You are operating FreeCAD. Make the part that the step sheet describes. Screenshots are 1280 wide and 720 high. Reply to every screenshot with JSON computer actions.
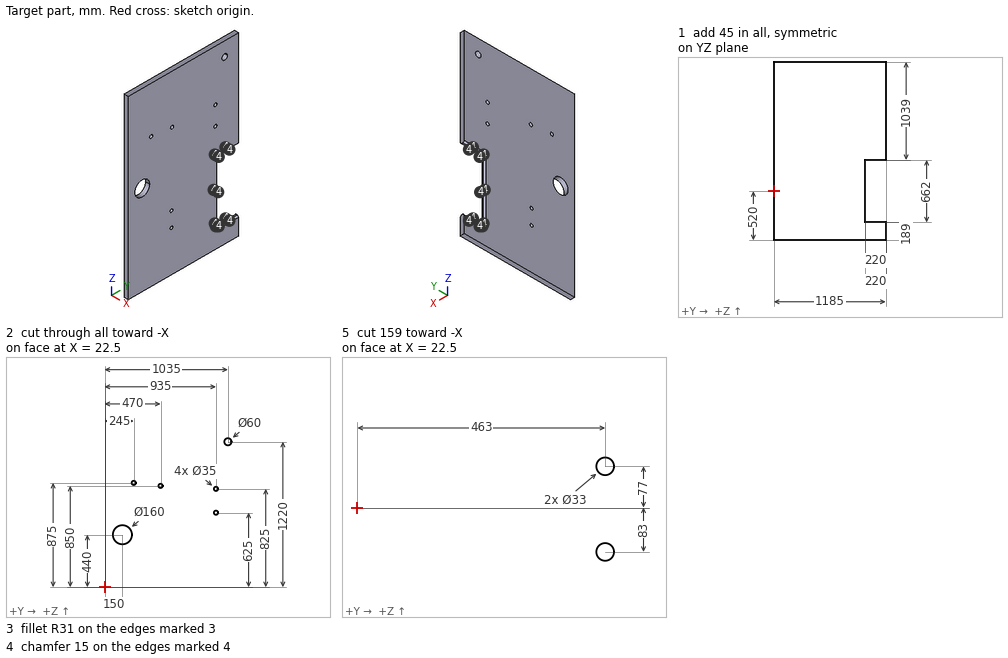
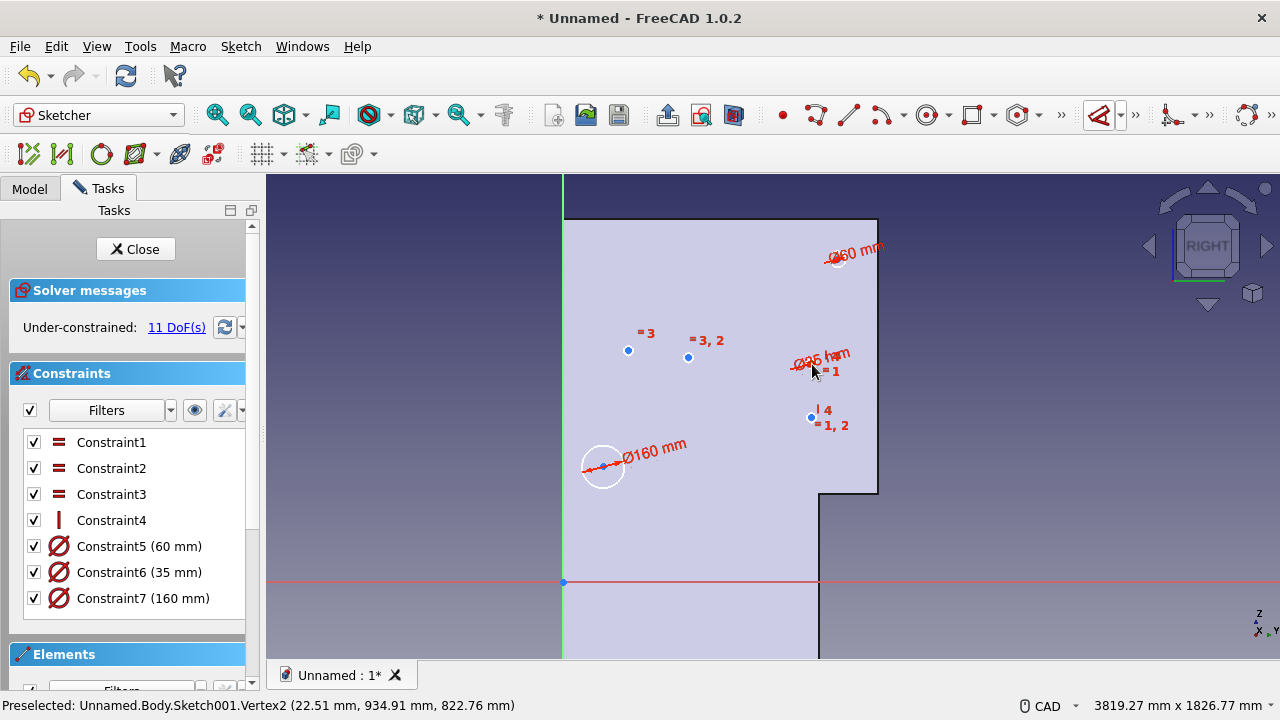
{"action": "left_click", "coordinate": [1120, 116]}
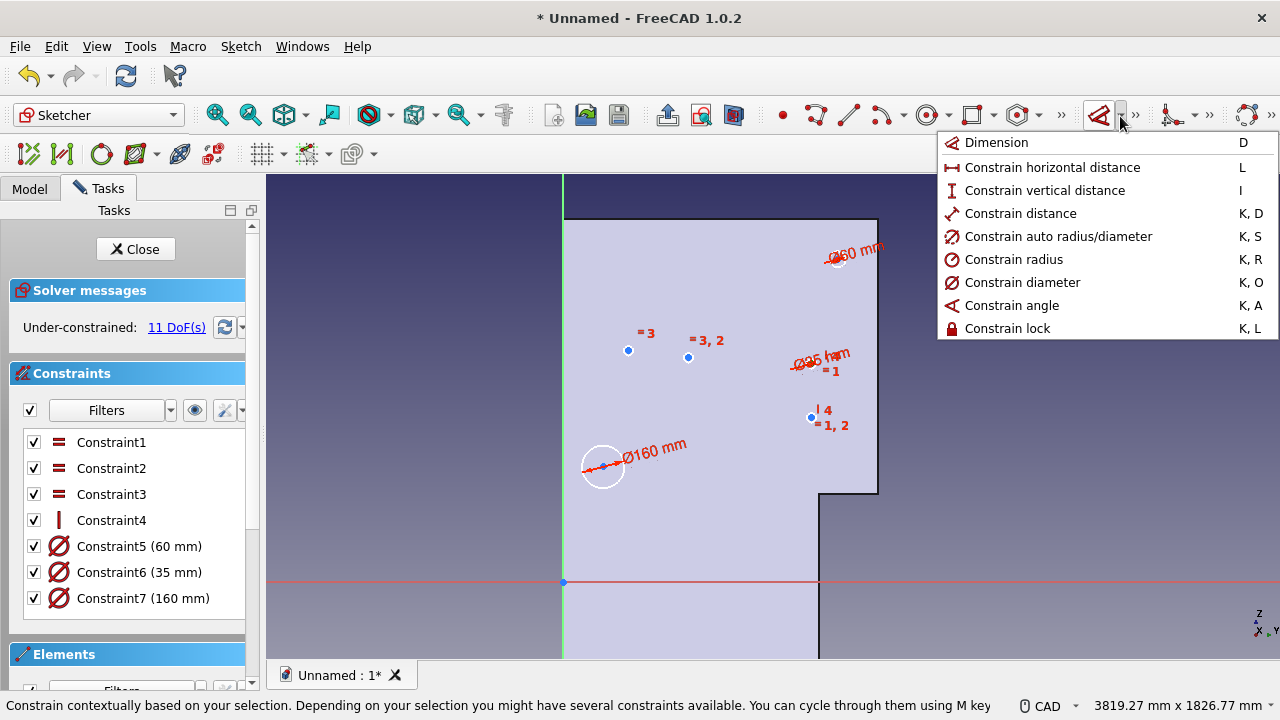
{"action": "left_click", "coordinate": [1108, 168]}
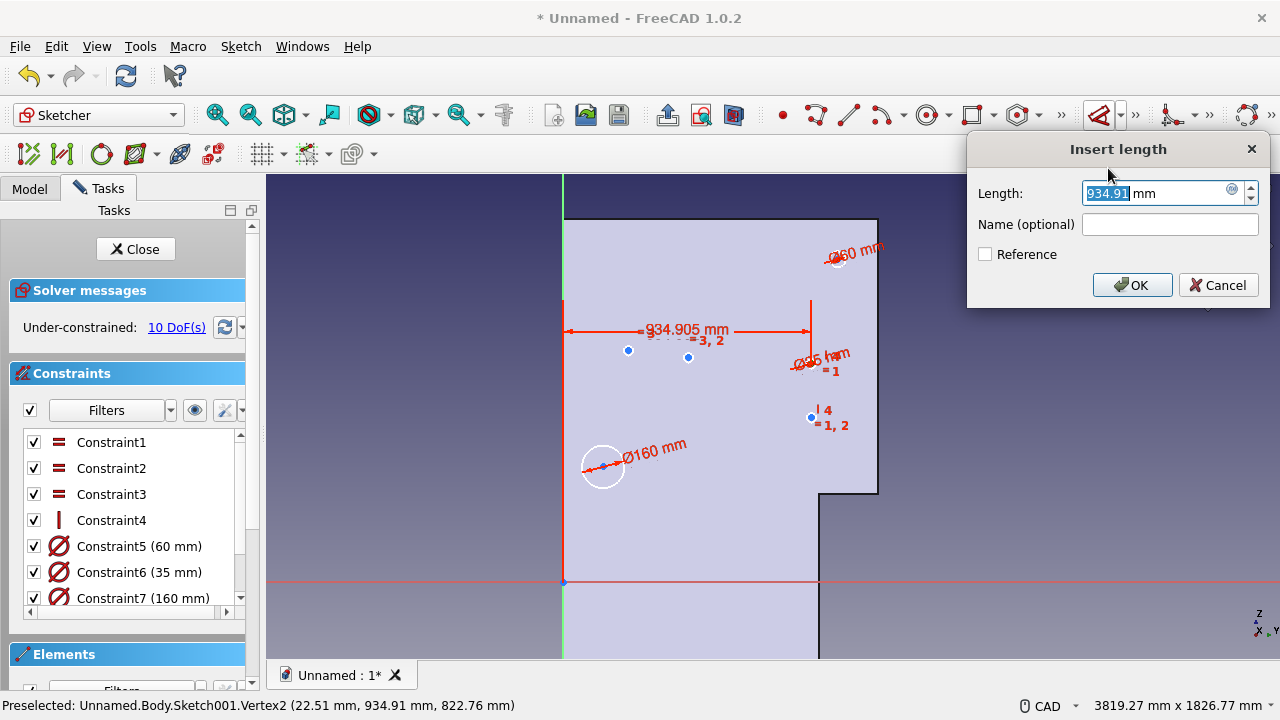
{"action": "type", "text": "935"}
{"action": "key", "text": "Return"}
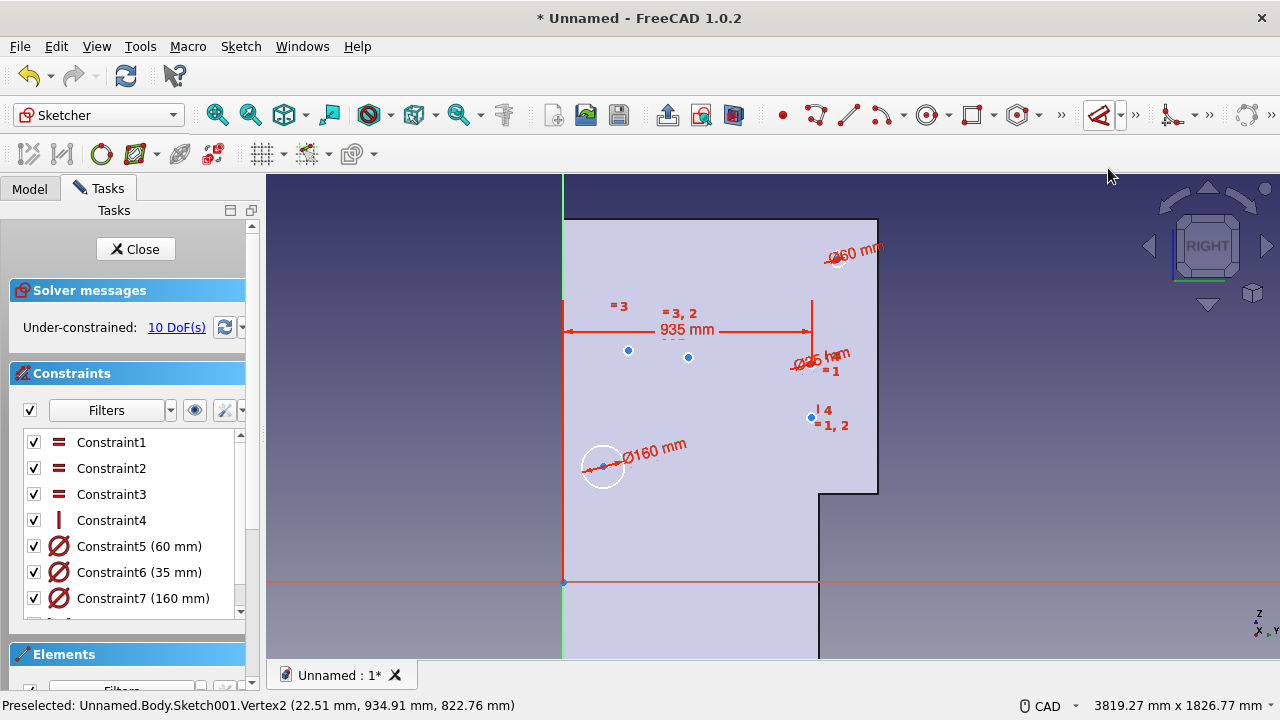
{"action": "left_click", "coordinate": [812, 364]}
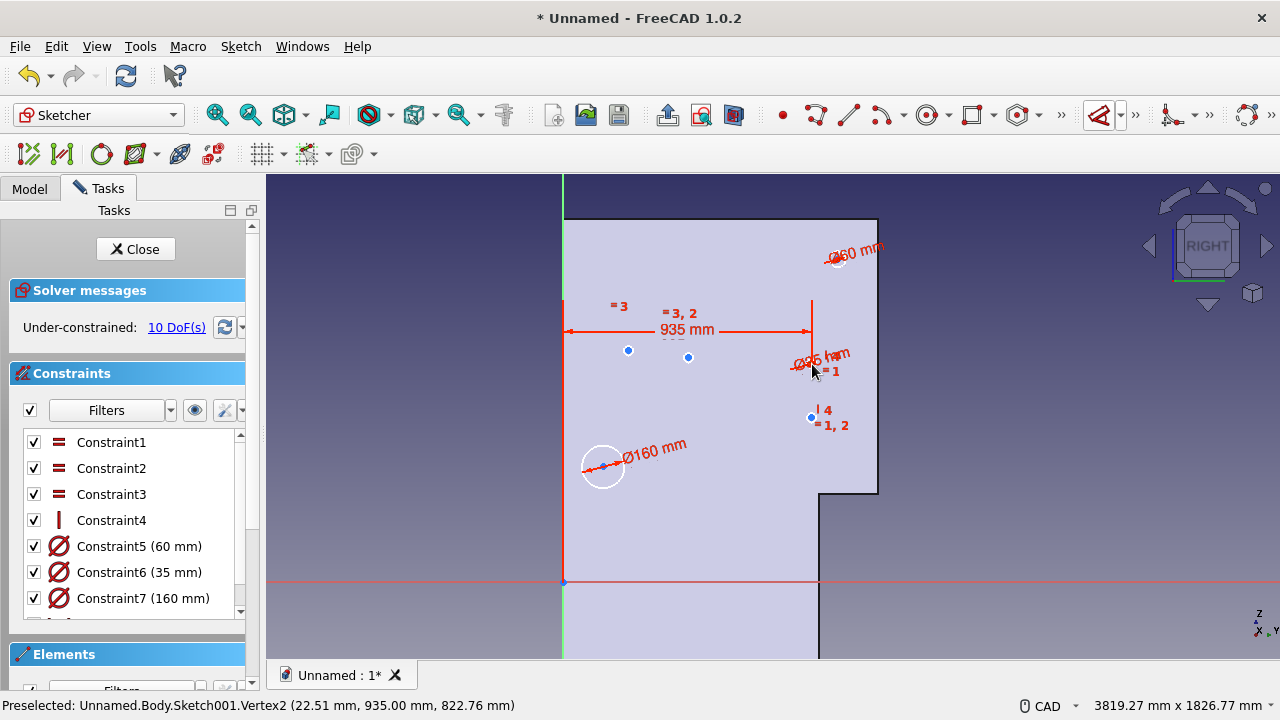
{"action": "key", "text": "i"}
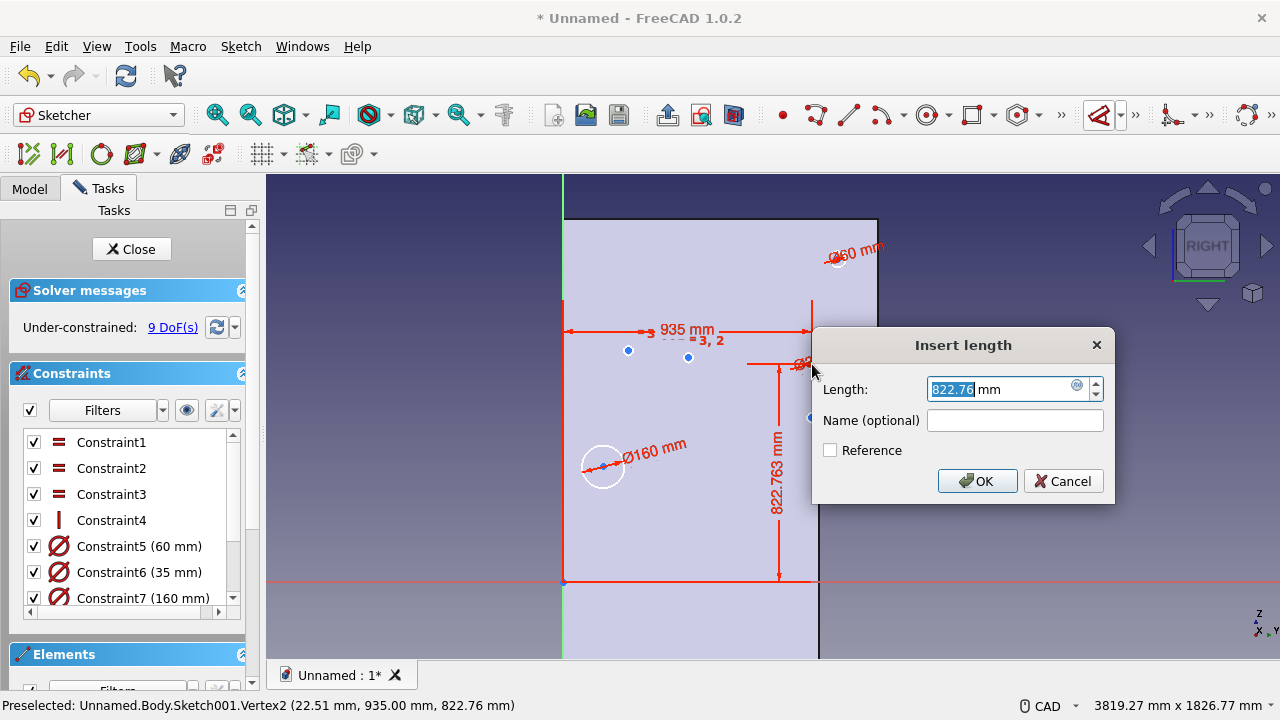
{"action": "type", "text": "825"}
{"action": "key", "text": "Return"}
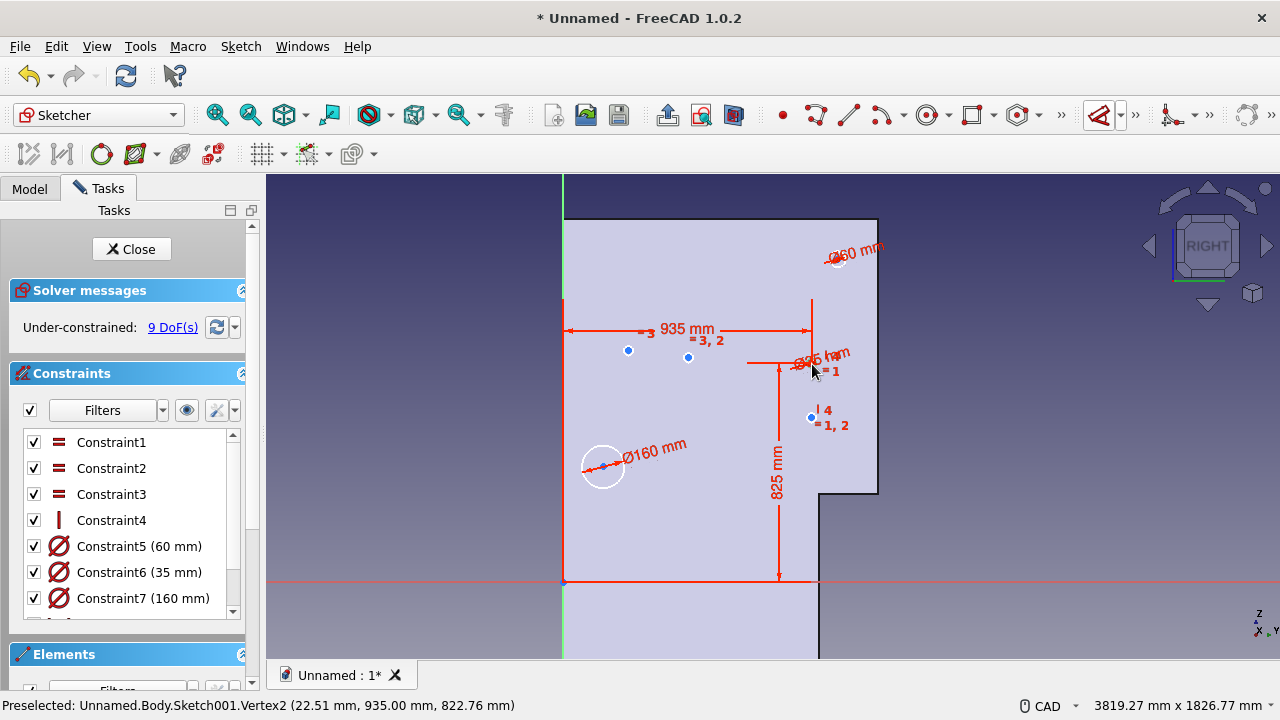
{"action": "left_click", "coordinate": [812, 418]}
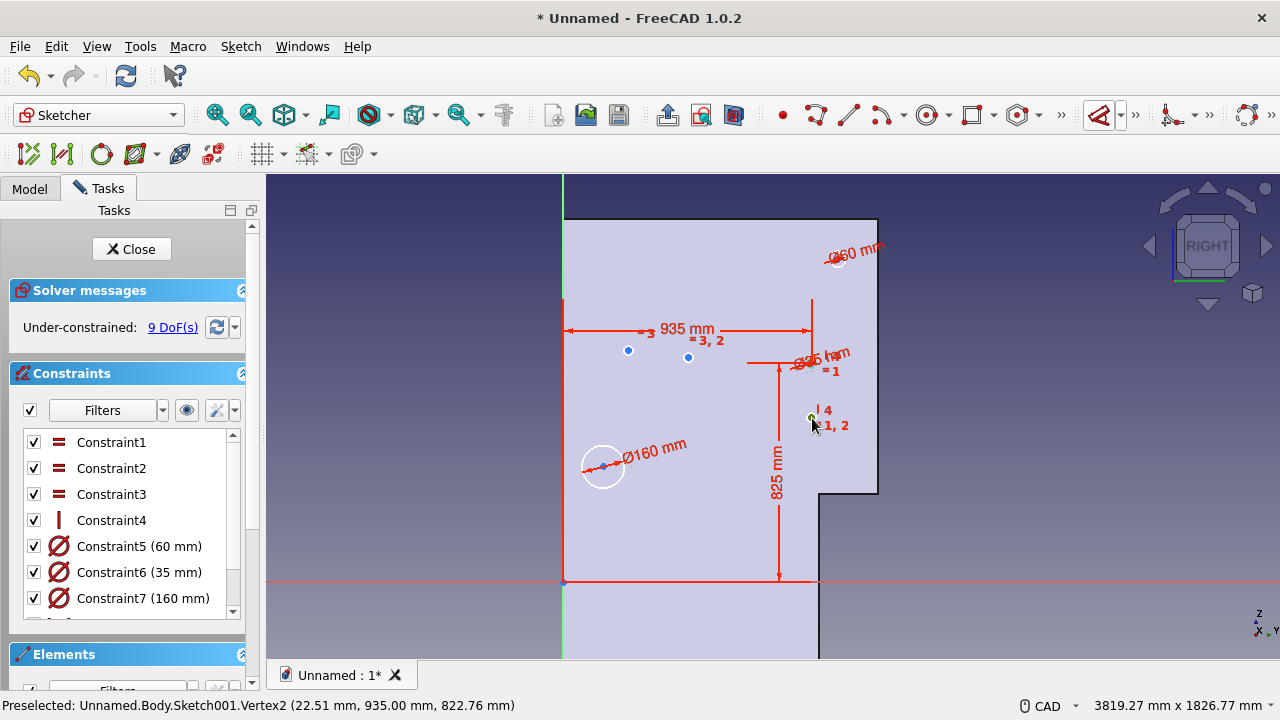
{"action": "key", "text": "i"}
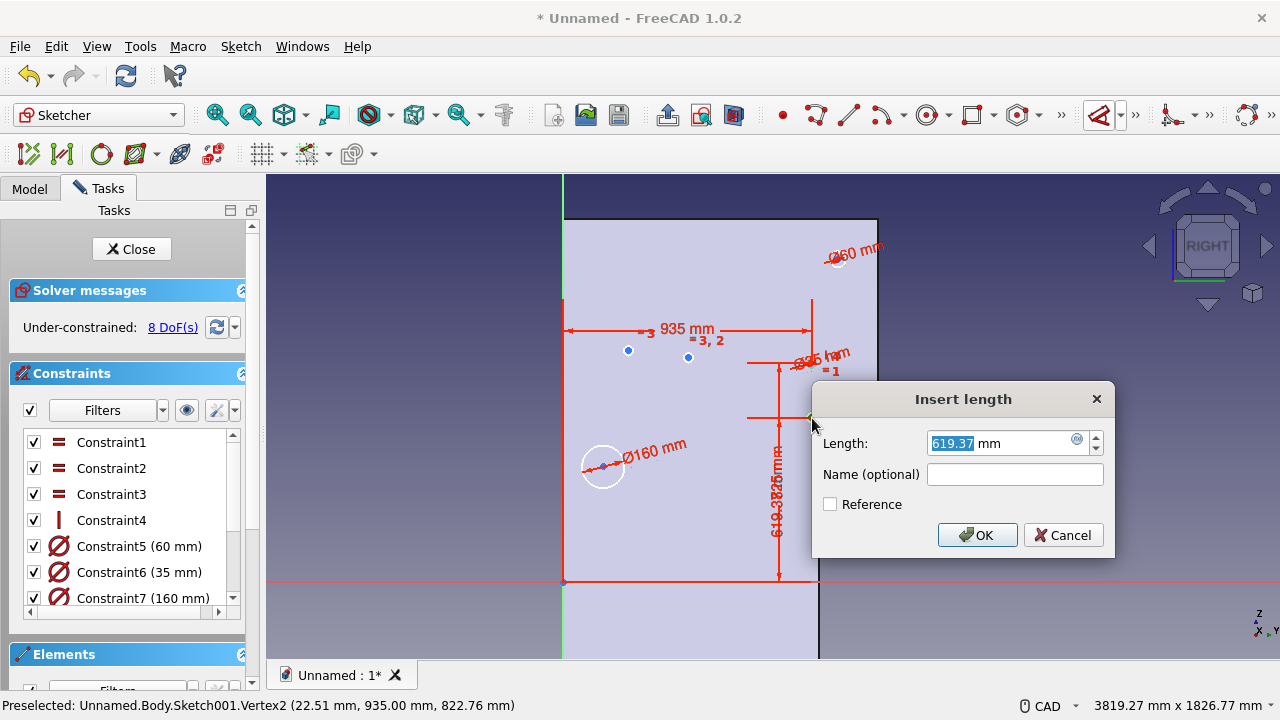
{"action": "type", "text": "625"}
{"action": "key", "text": "Return"}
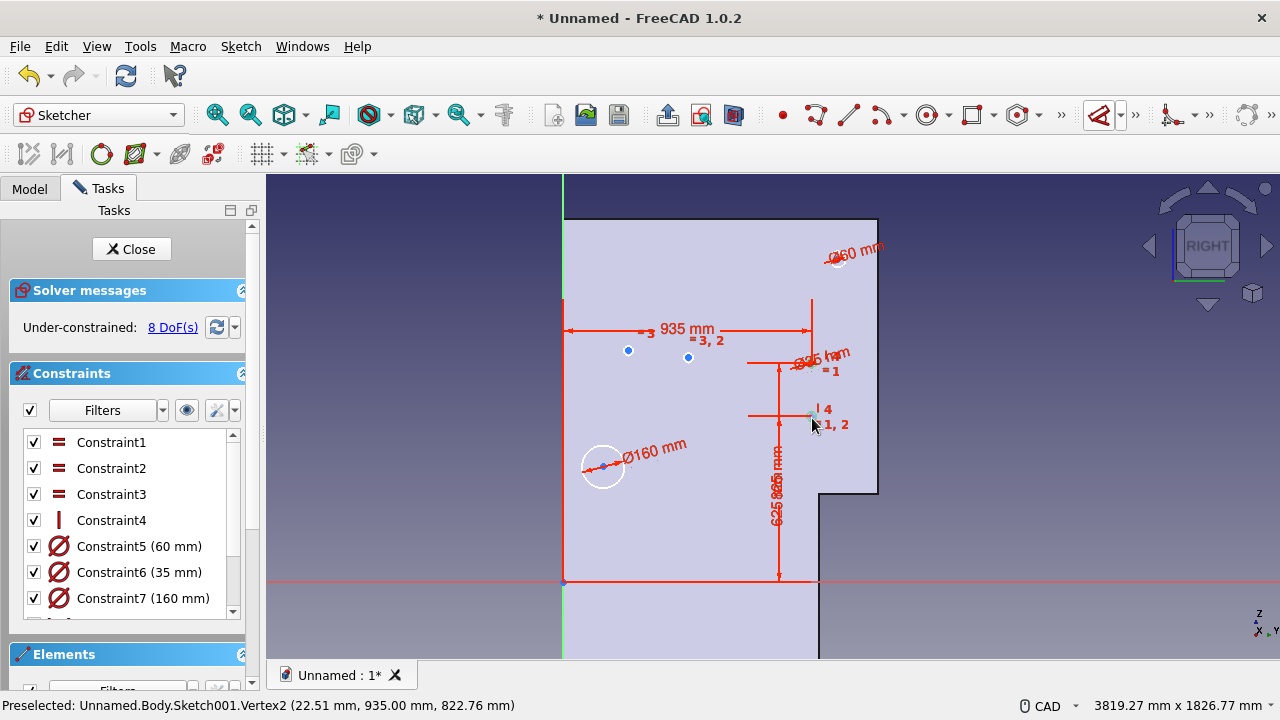
{"action": "left_click", "coordinate": [689, 358]}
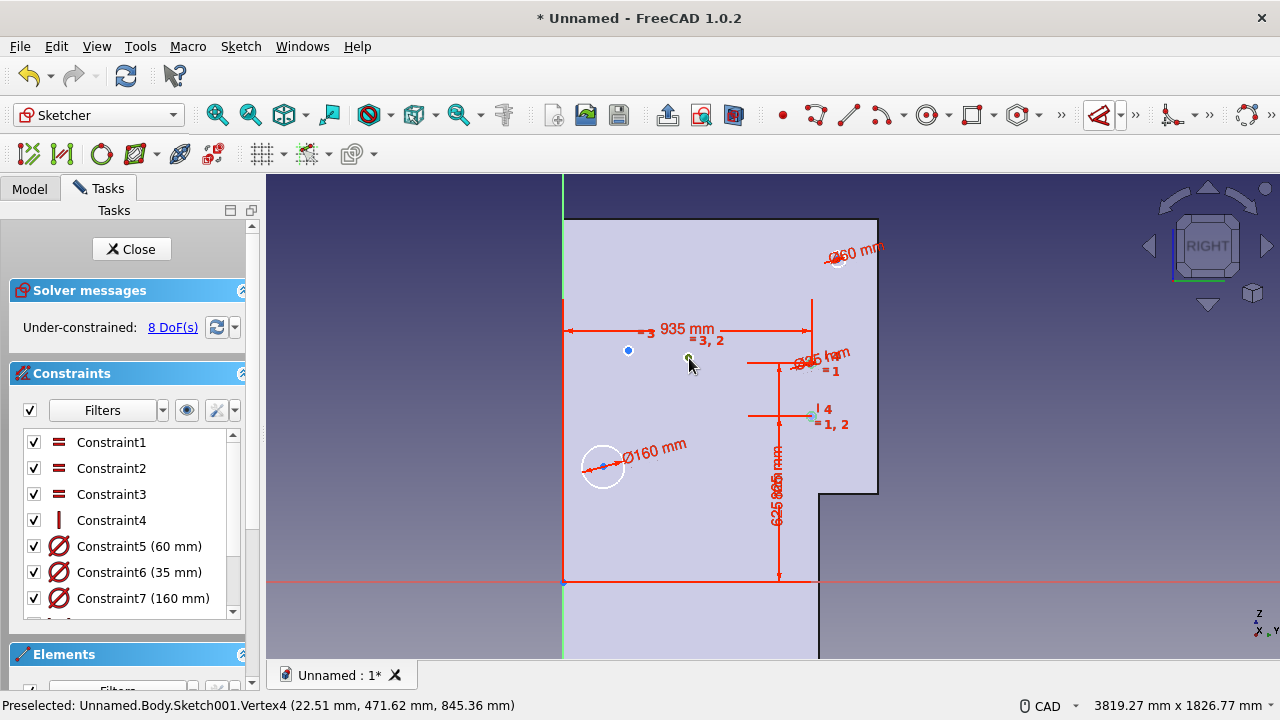
{"action": "left_click", "coordinate": [1120, 116]}